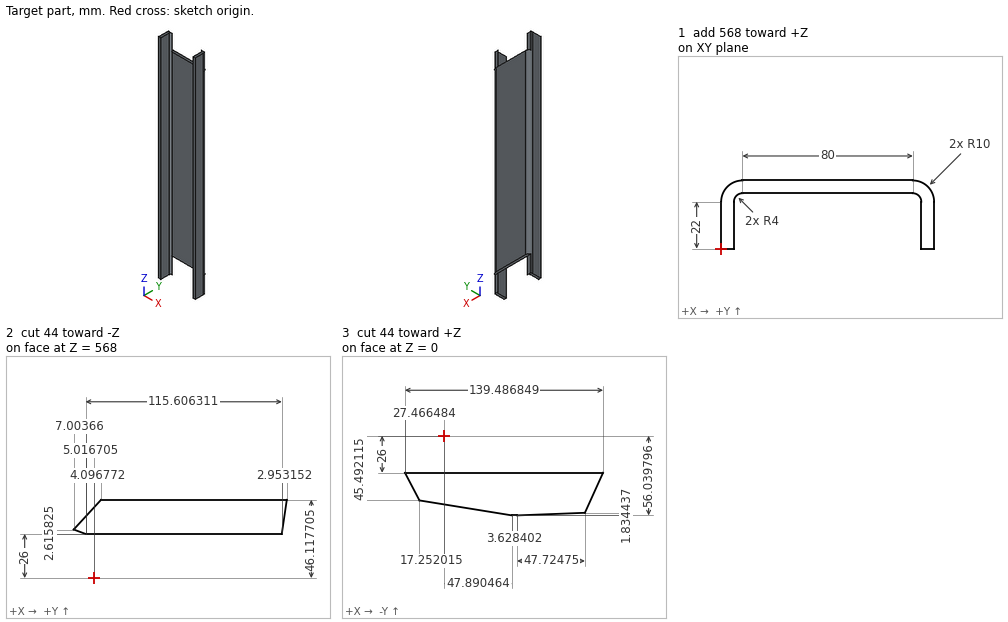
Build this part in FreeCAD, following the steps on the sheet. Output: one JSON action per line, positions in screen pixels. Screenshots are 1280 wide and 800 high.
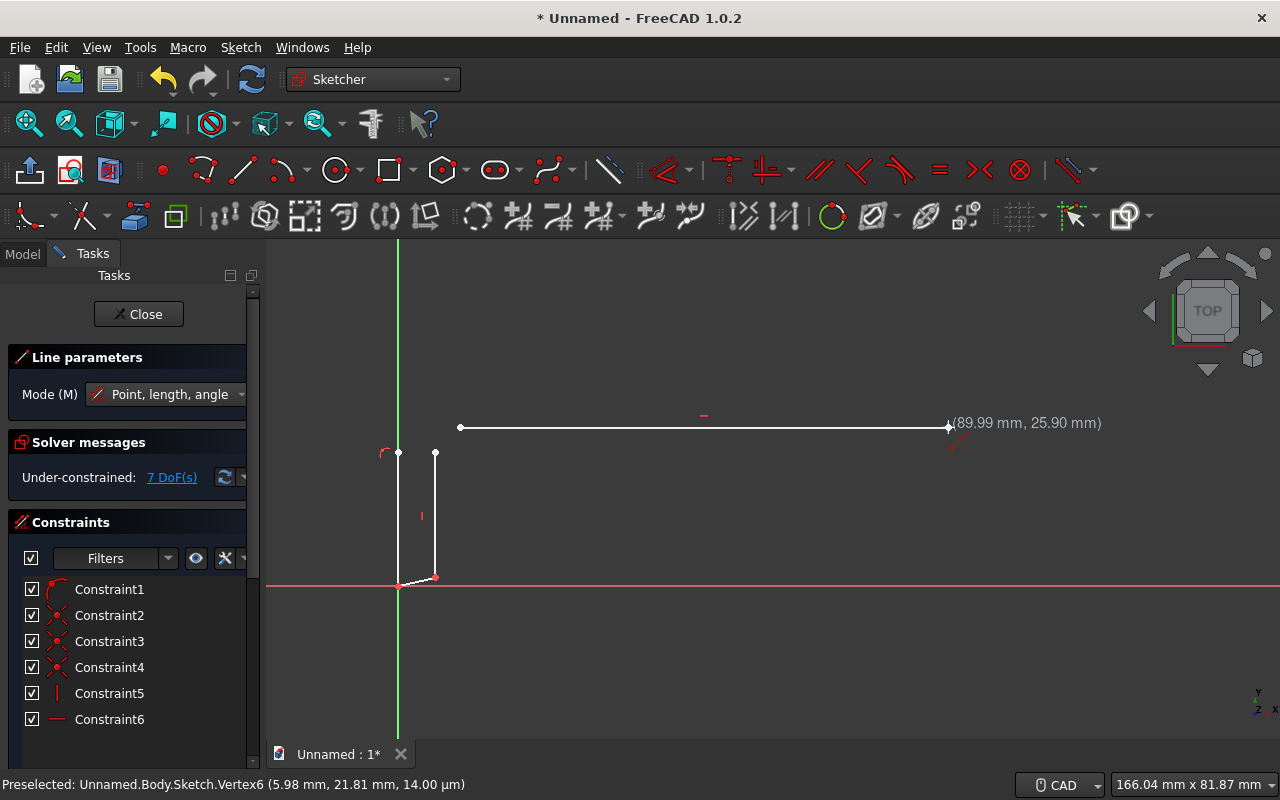
{"action": "left_click", "coordinate": [204, 170]}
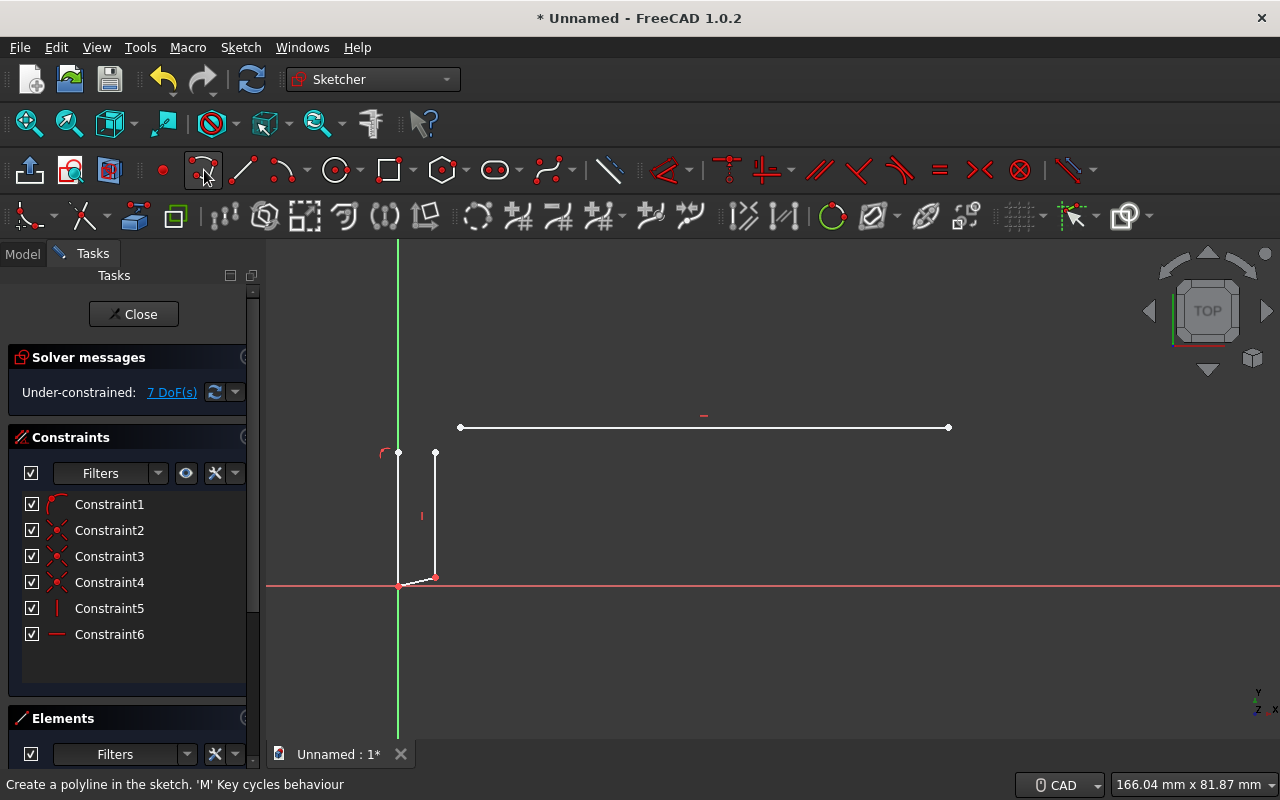
{"action": "left_click", "coordinate": [973, 452]}
{"action": "left_click", "coordinate": [973, 586]}
{"action": "left_click", "coordinate": [1009, 577]}
{"action": "left_click", "coordinate": [1009, 452]}
{"action": "right_click", "coordinate": [1009, 452]}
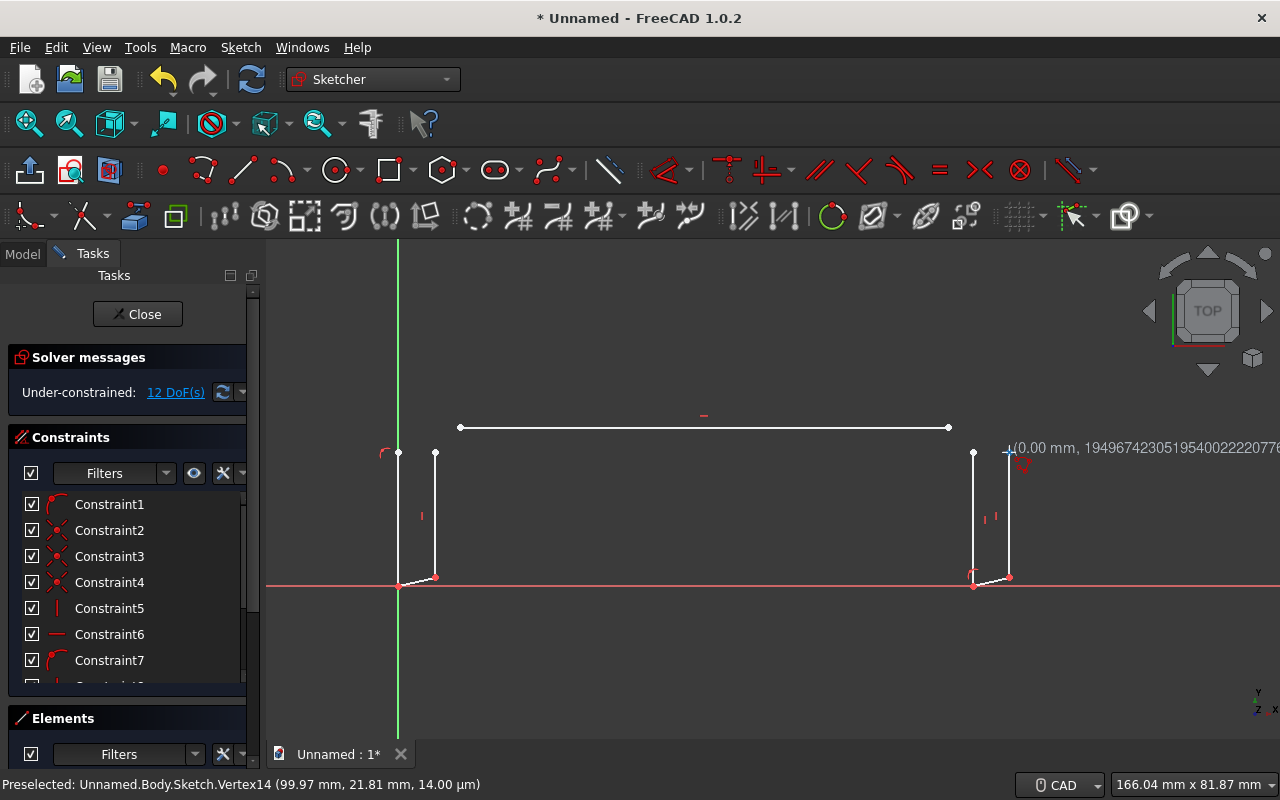
{"action": "left_click", "coordinate": [244, 170]}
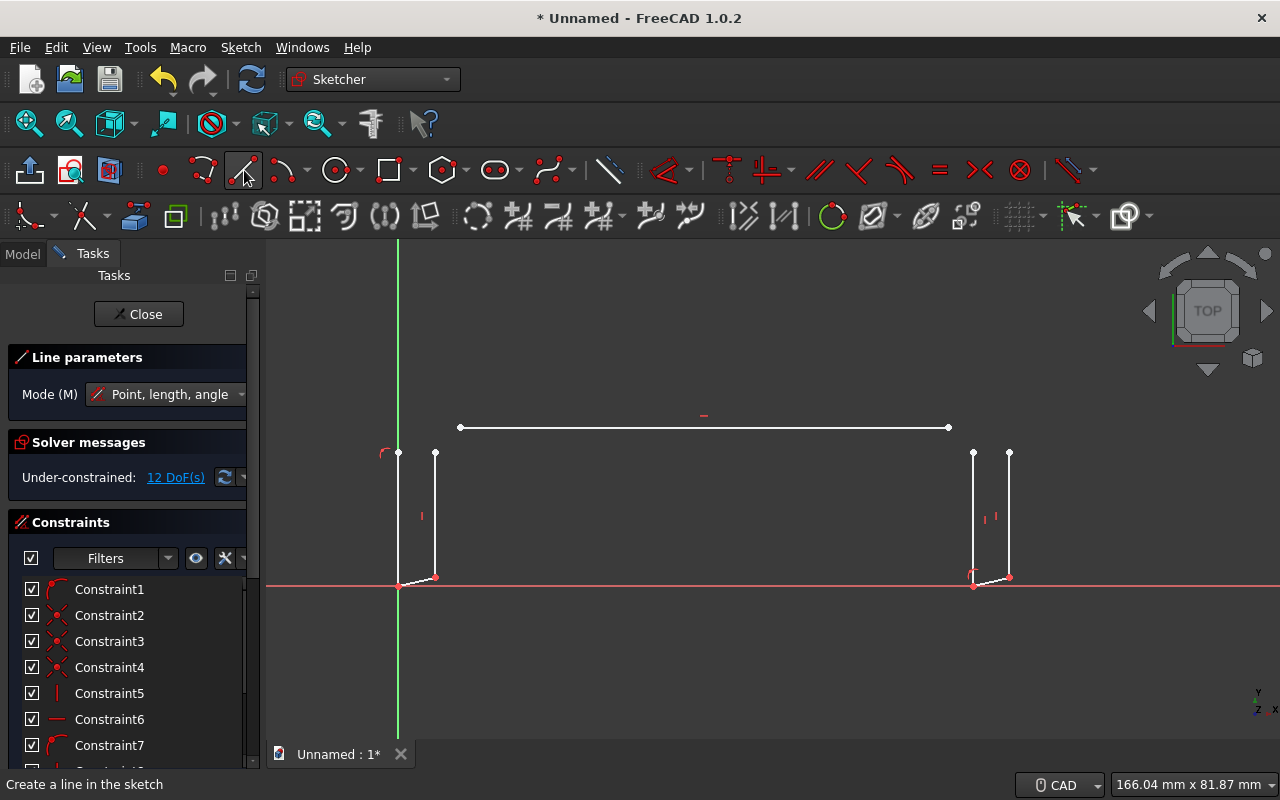
{"action": "left_click", "coordinate": [948, 391]}
{"action": "left_click", "coordinate": [460, 391]}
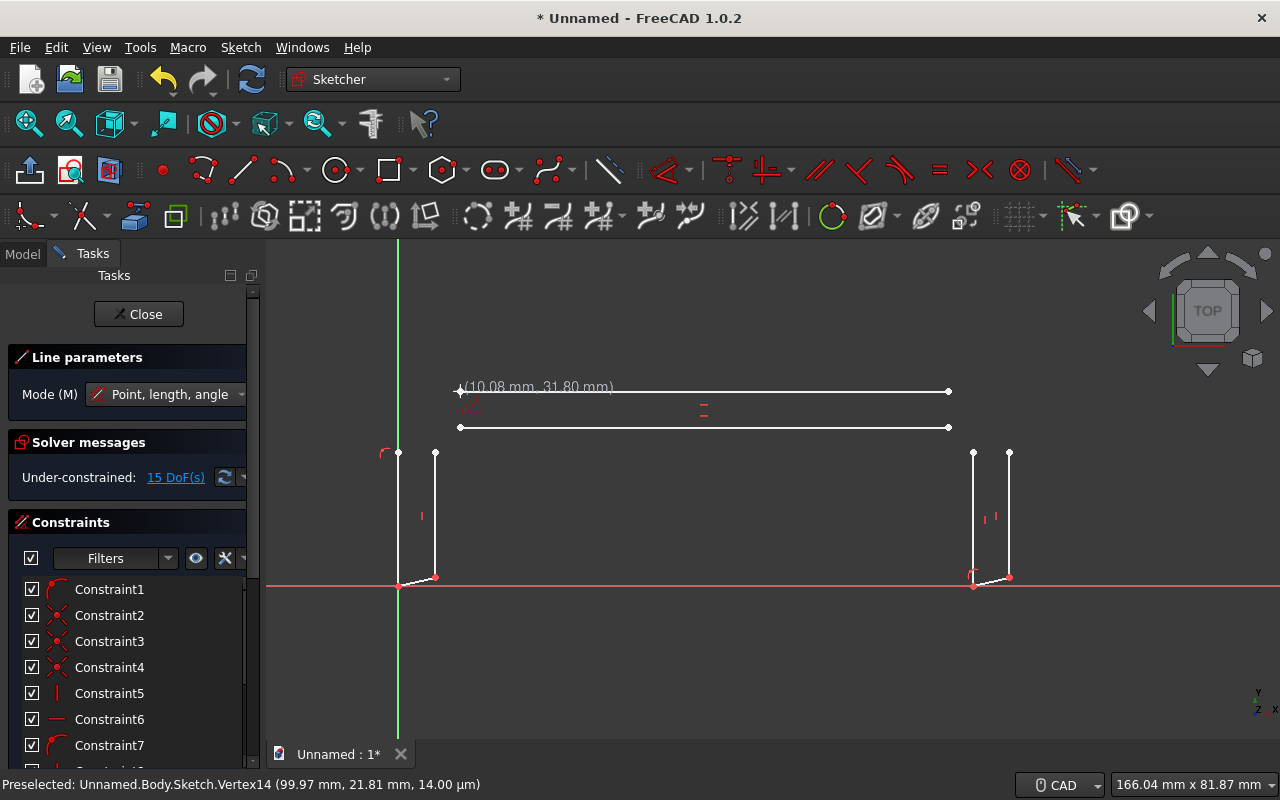
{"action": "left_click", "coordinate": [310, 170]}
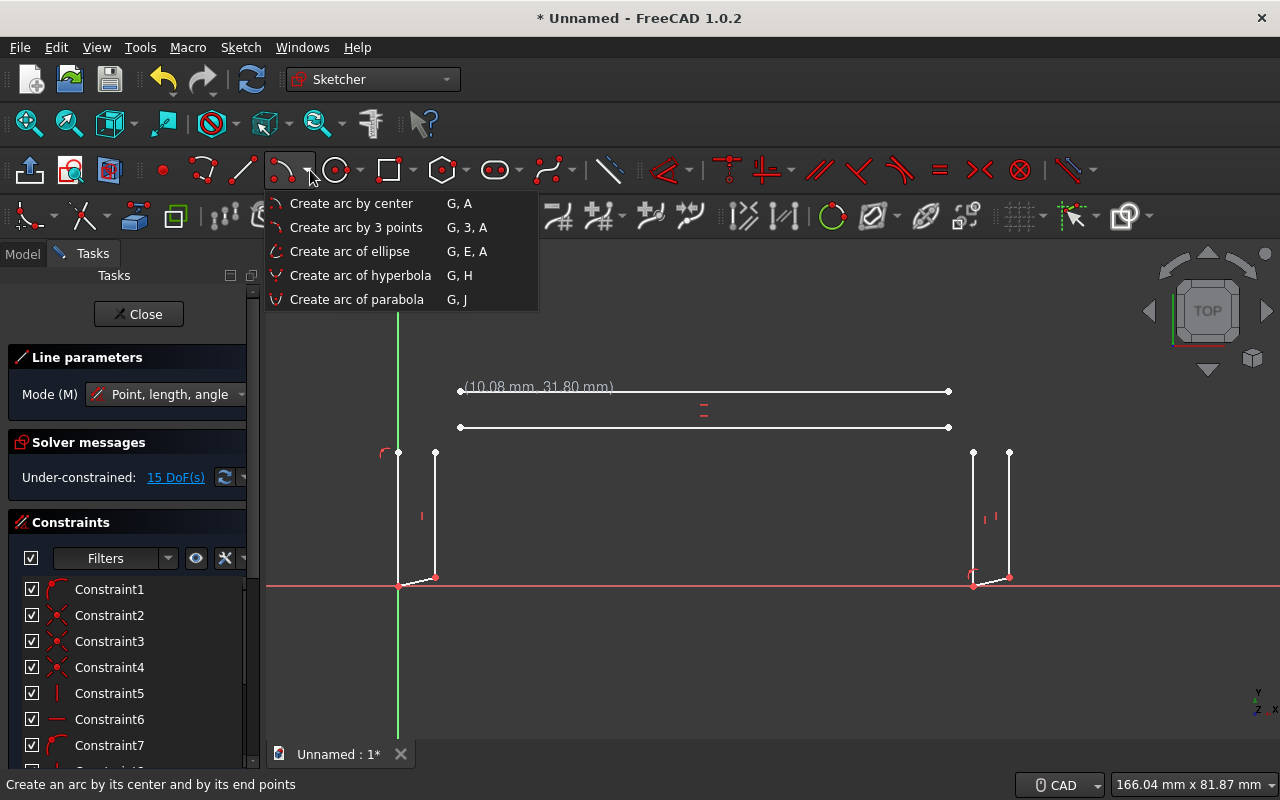
{"action": "left_click", "coordinate": [402, 227]}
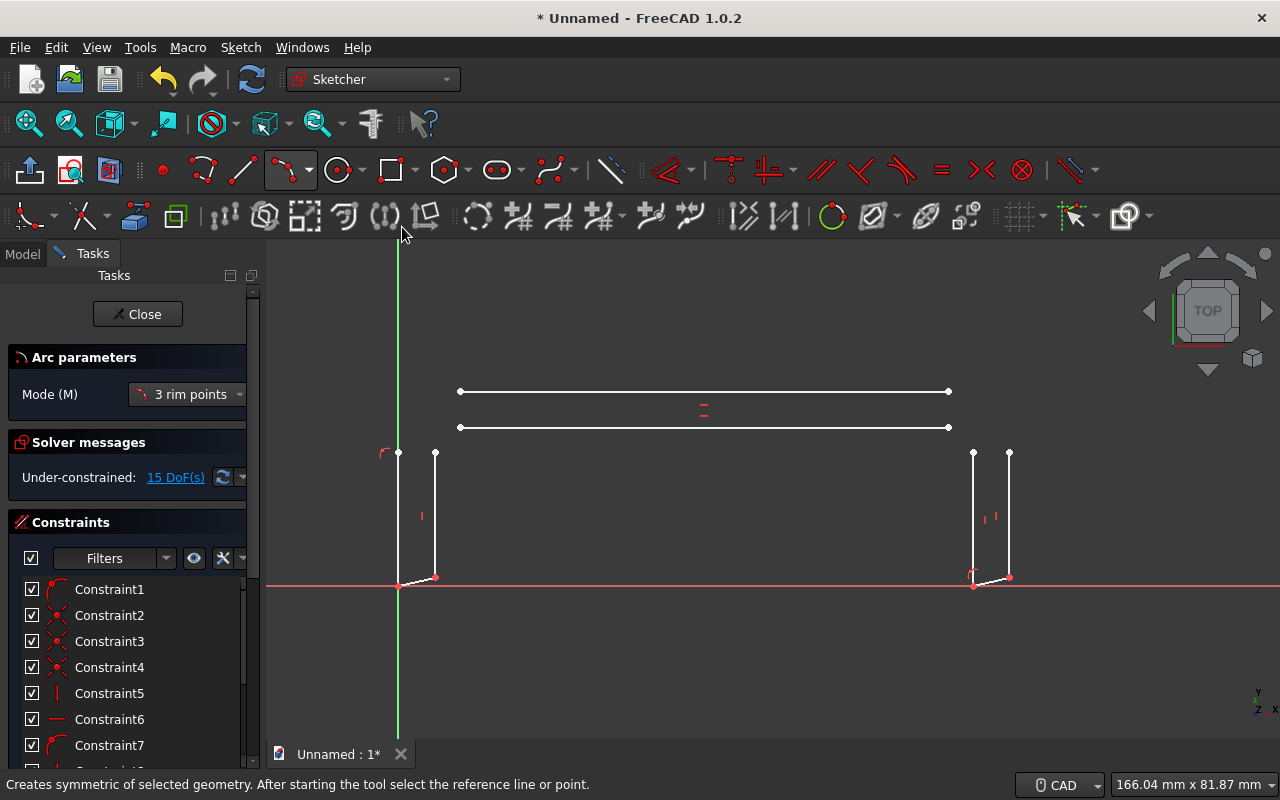
{"action": "left_click", "coordinate": [435, 453]}
{"action": "left_click", "coordinate": [460, 428]}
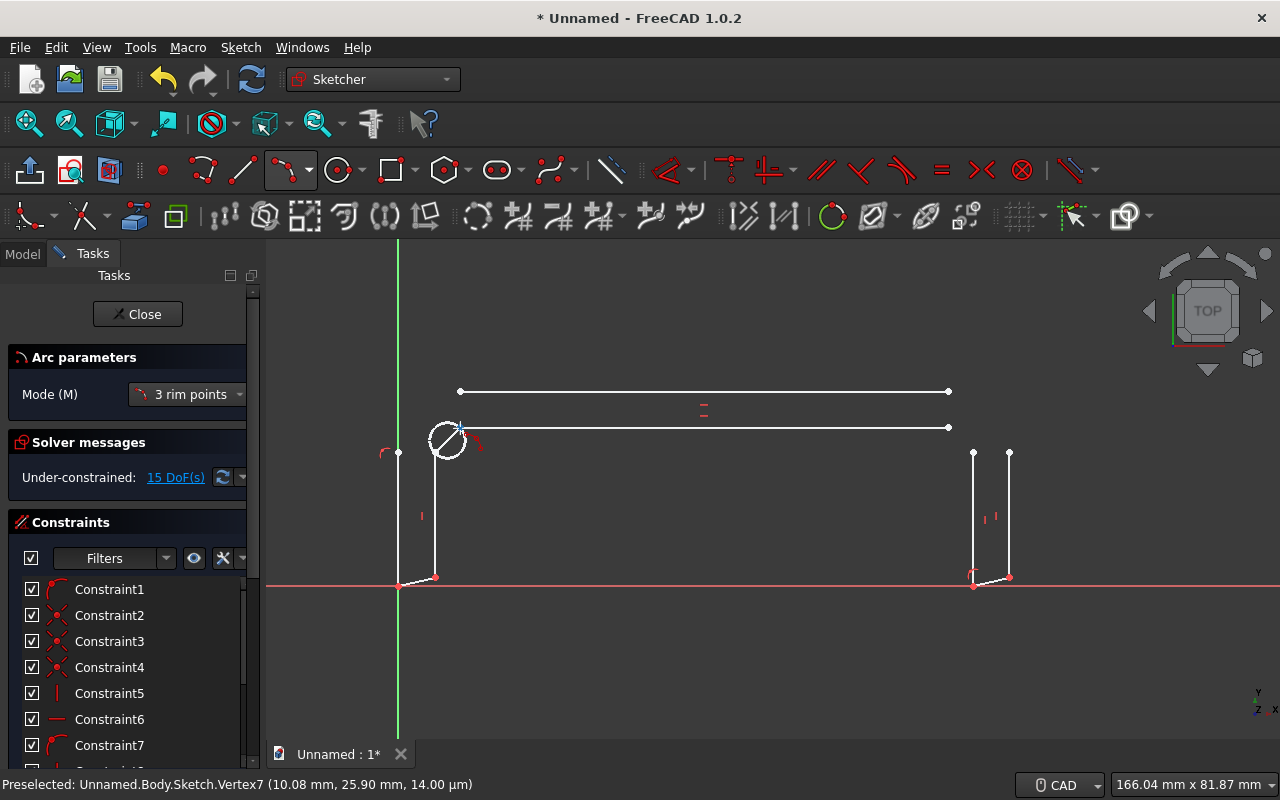
{"action": "scroll", "coordinate": [442, 435], "scroll_direction": "up", "scroll_amount": 4}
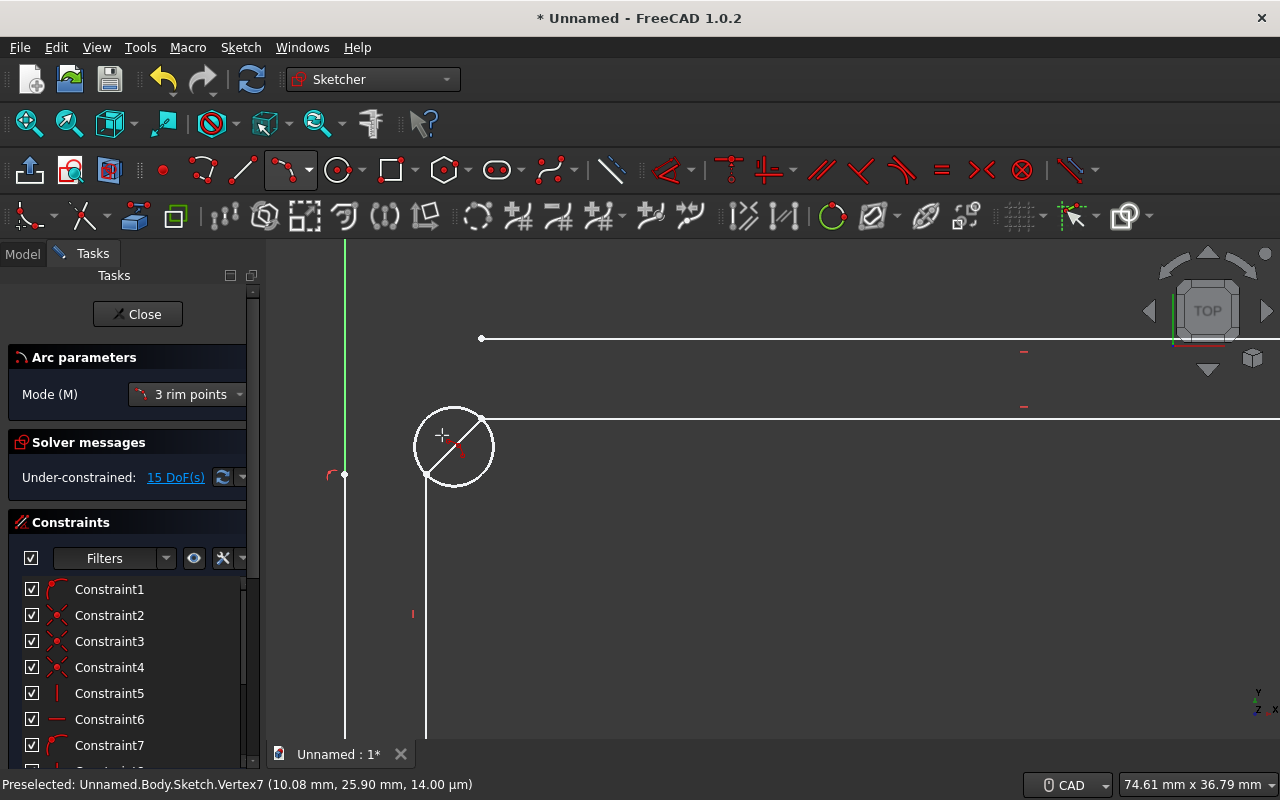
{"action": "left_click", "coordinate": [442, 434]}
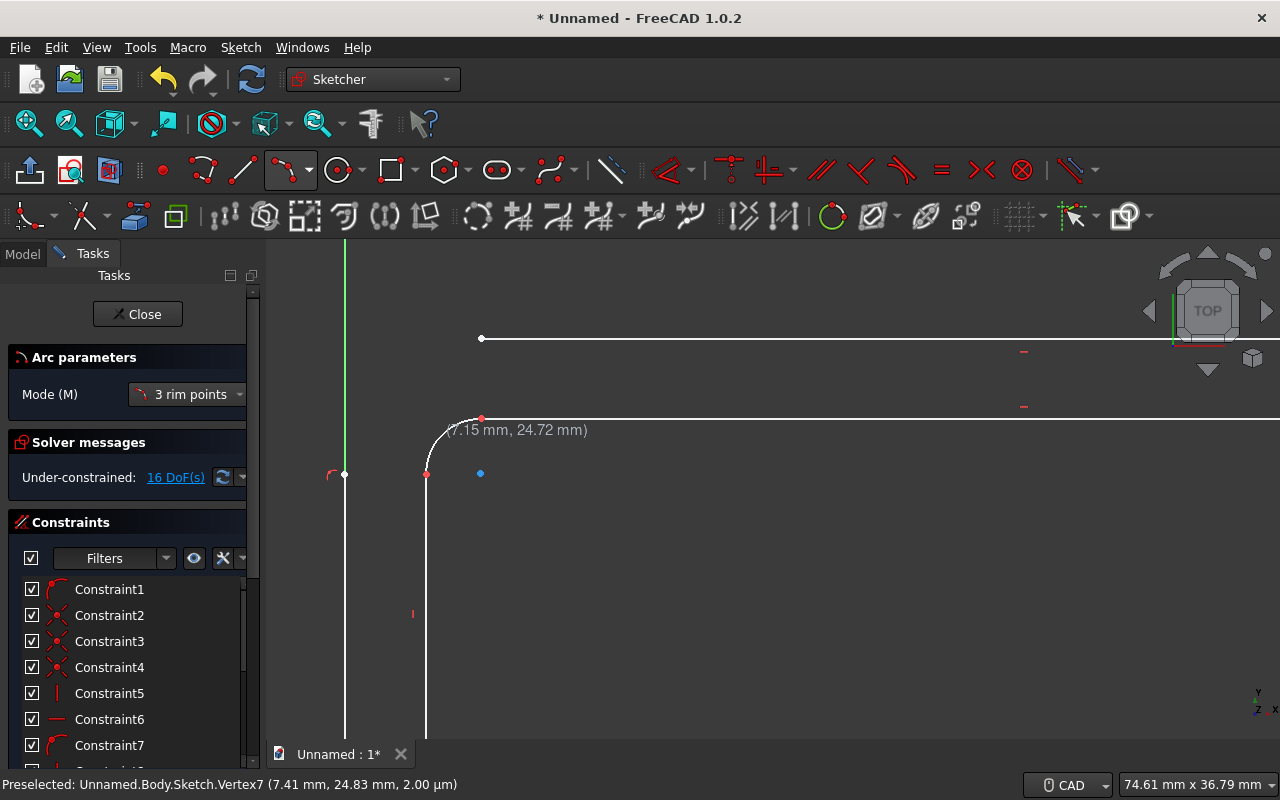
{"action": "scroll", "coordinate": [443, 436], "scroll_direction": "down", "scroll_amount": 4}